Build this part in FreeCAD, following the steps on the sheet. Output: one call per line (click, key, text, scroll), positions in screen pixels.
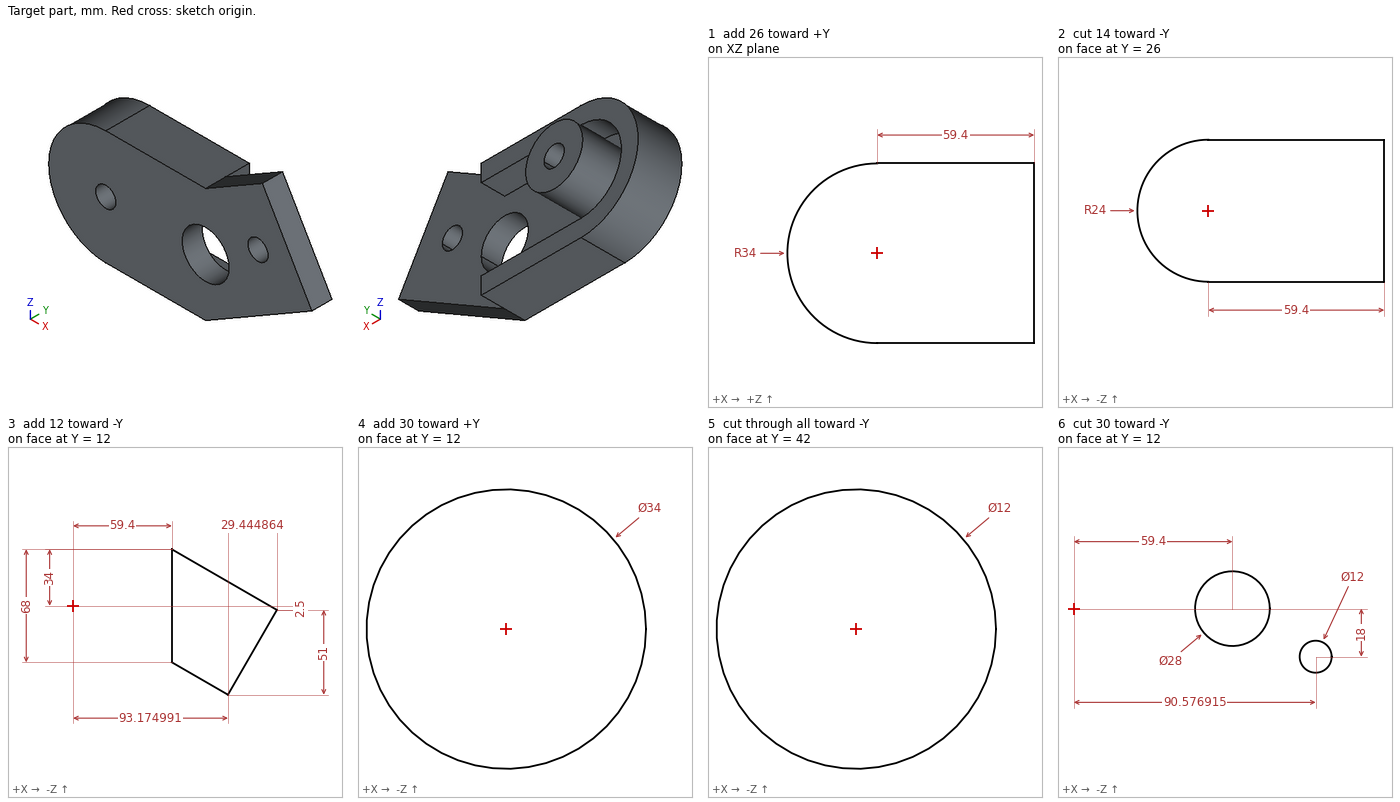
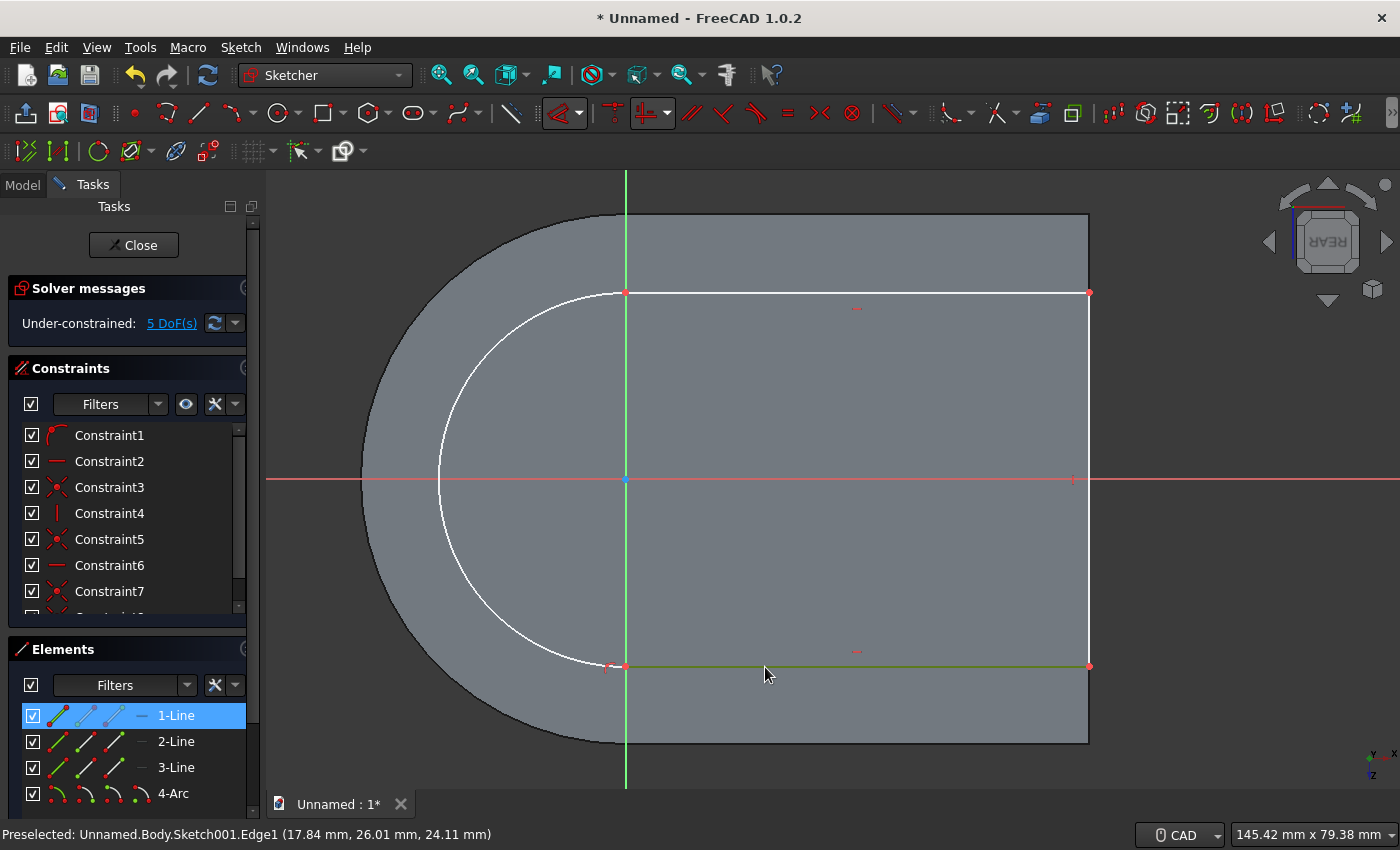
click(475, 370)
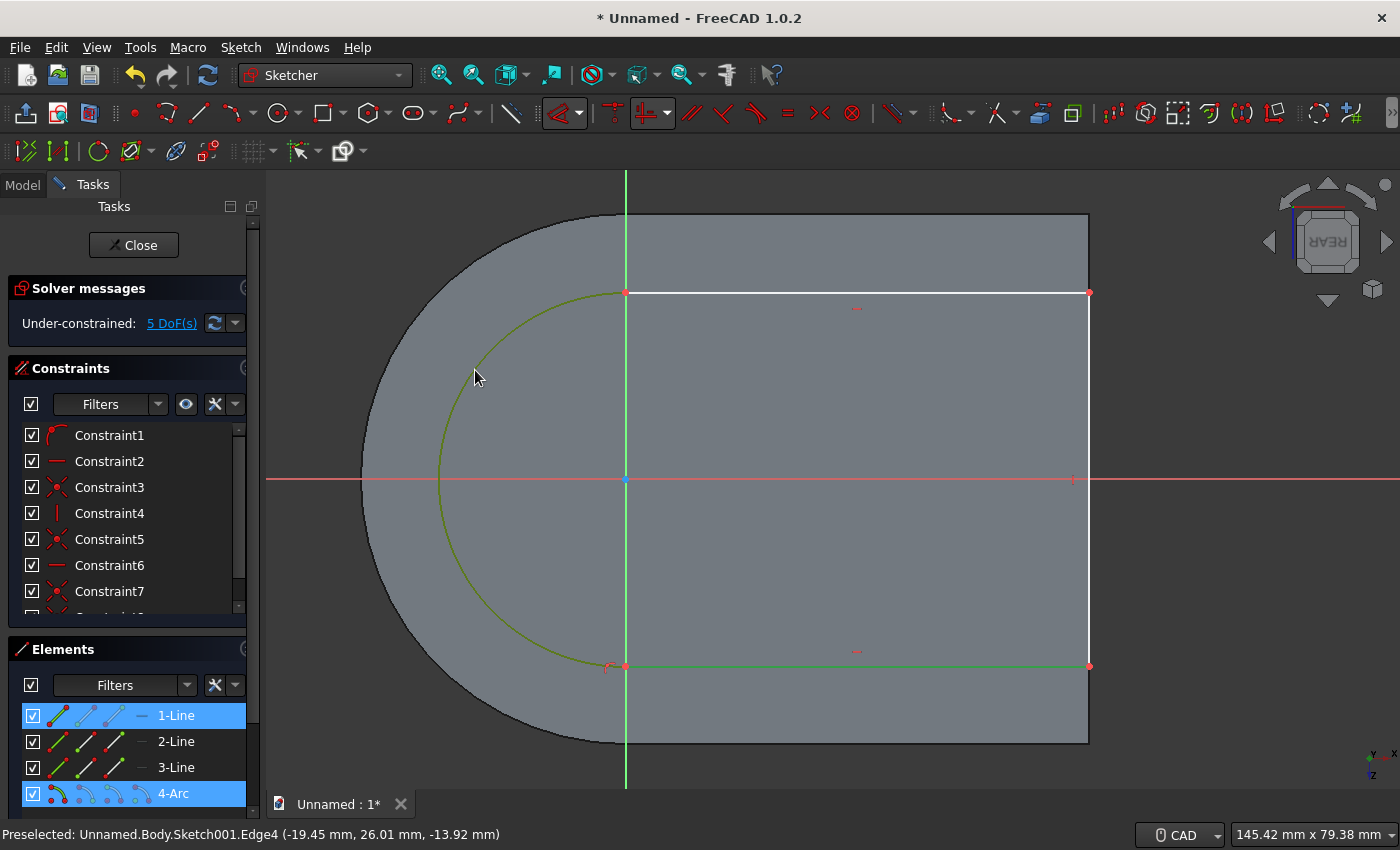
click(756, 114)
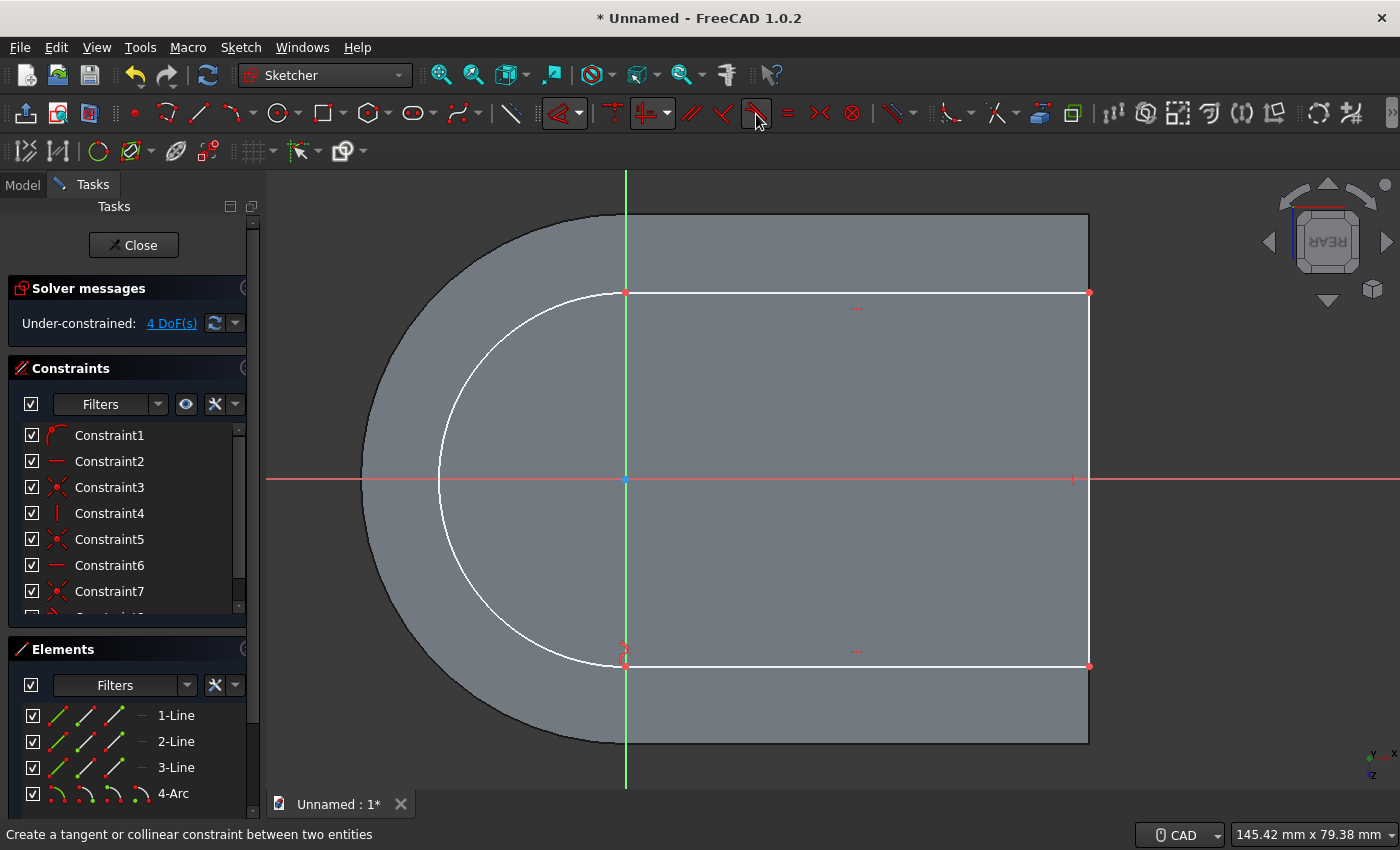
click(950, 293)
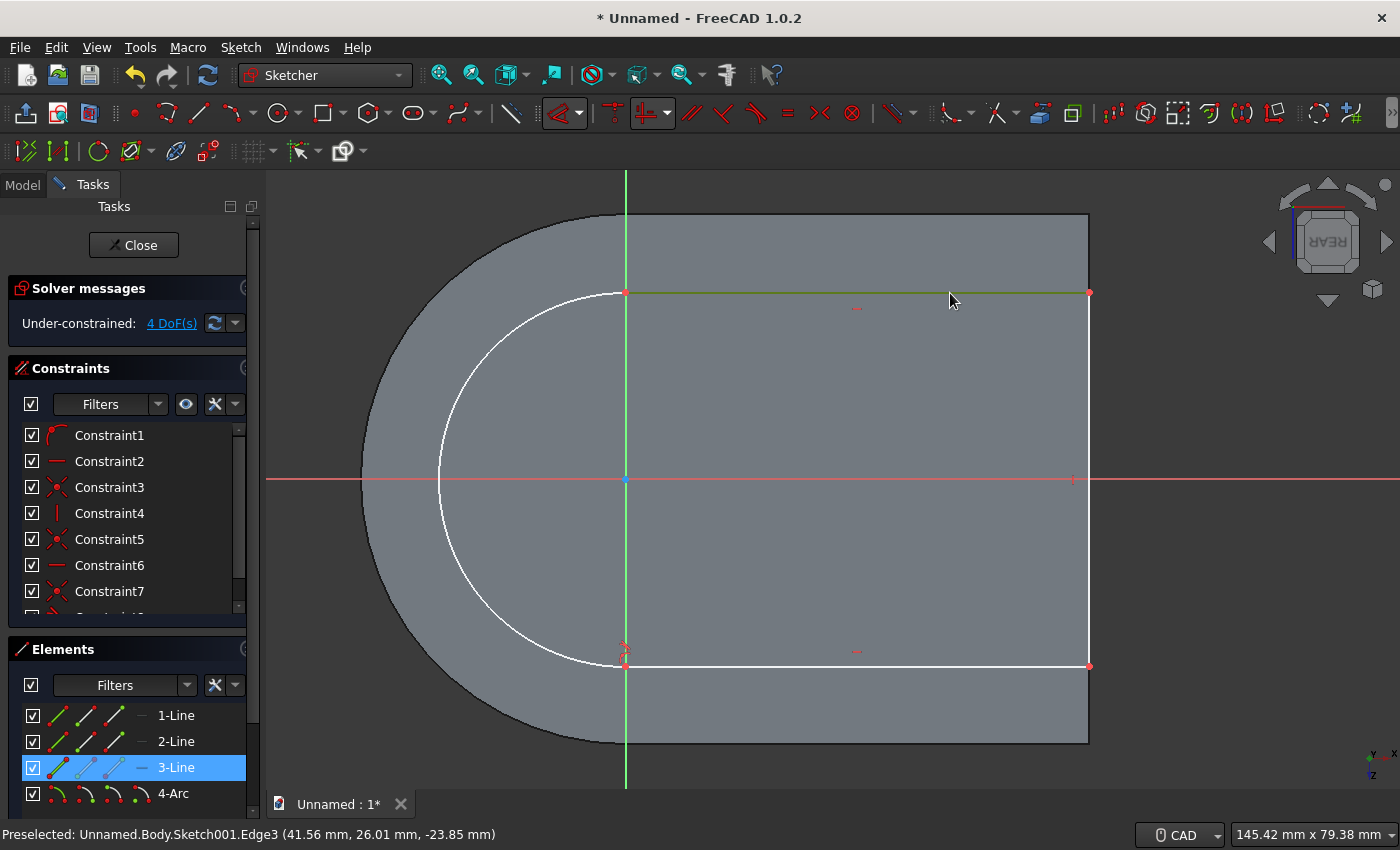
click(475, 370)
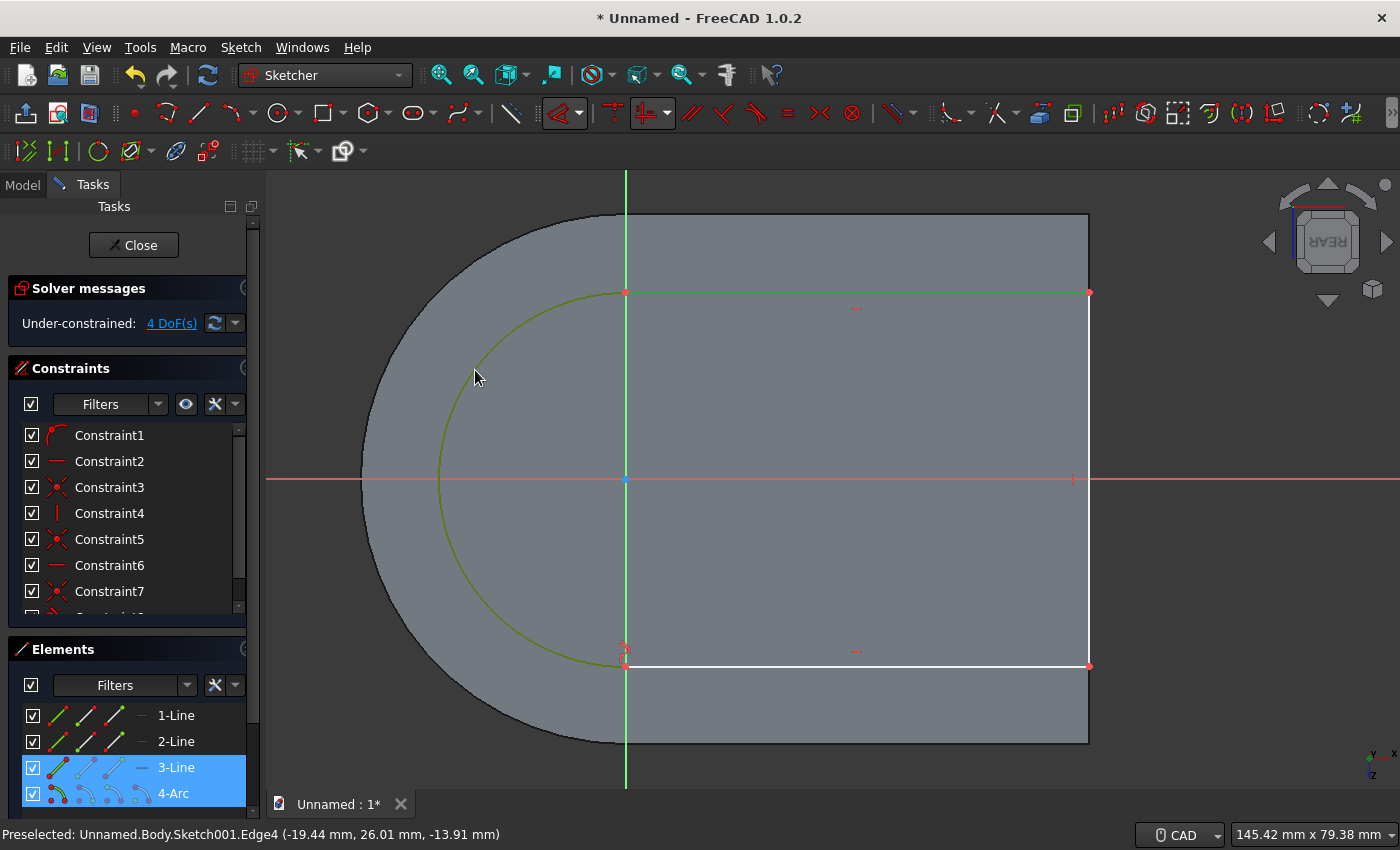
click(756, 114)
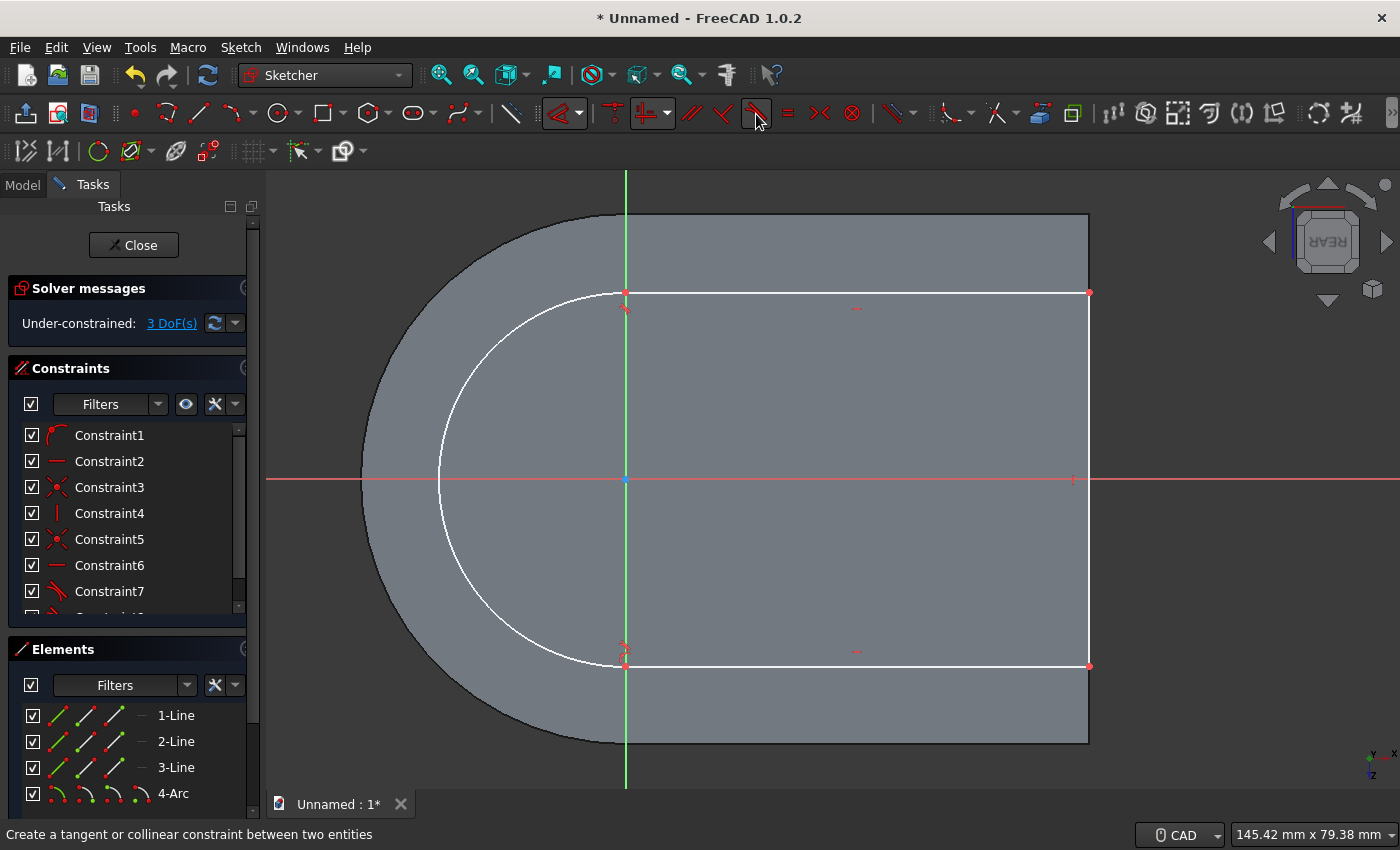
click(626, 480)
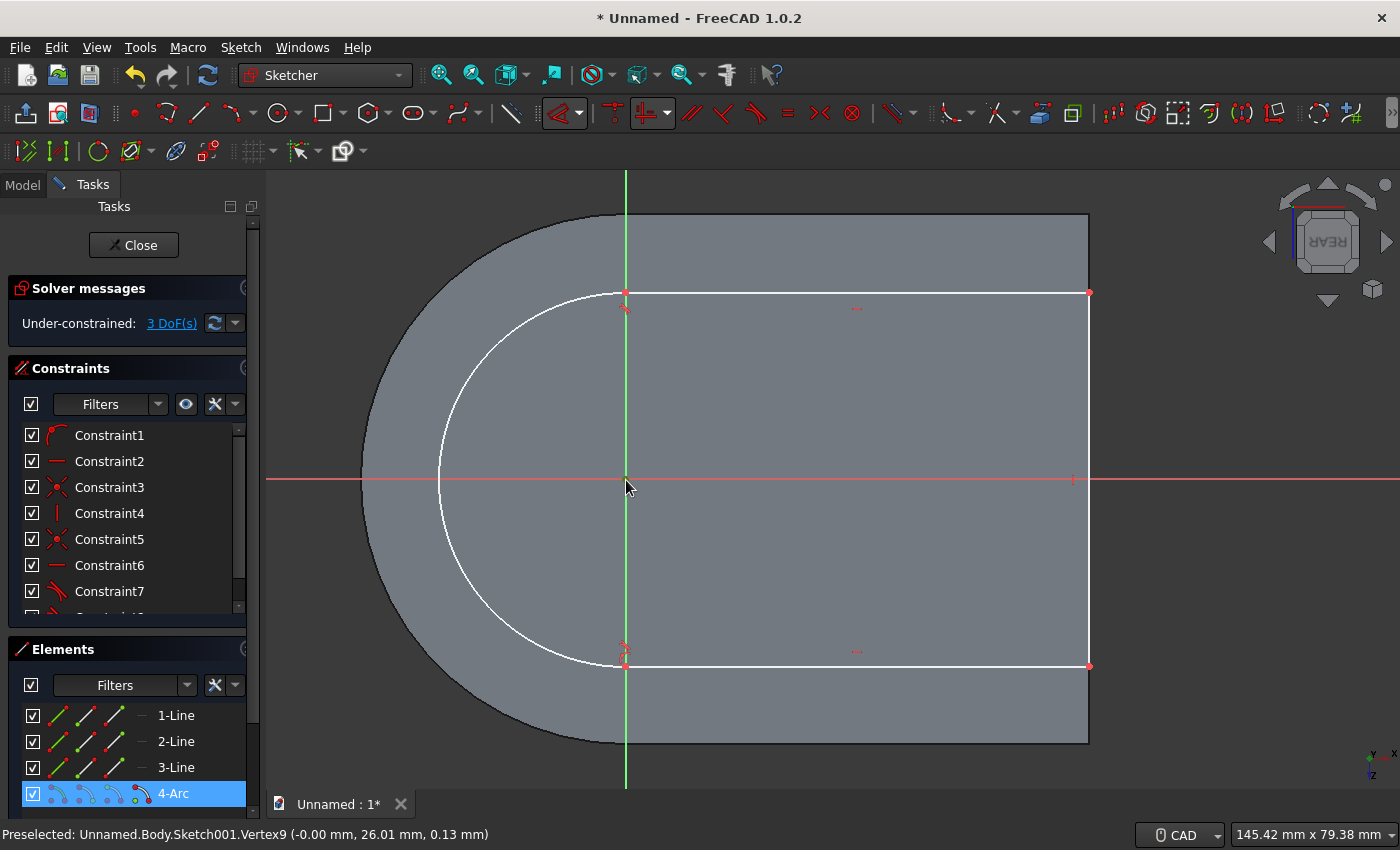
click(361, 479)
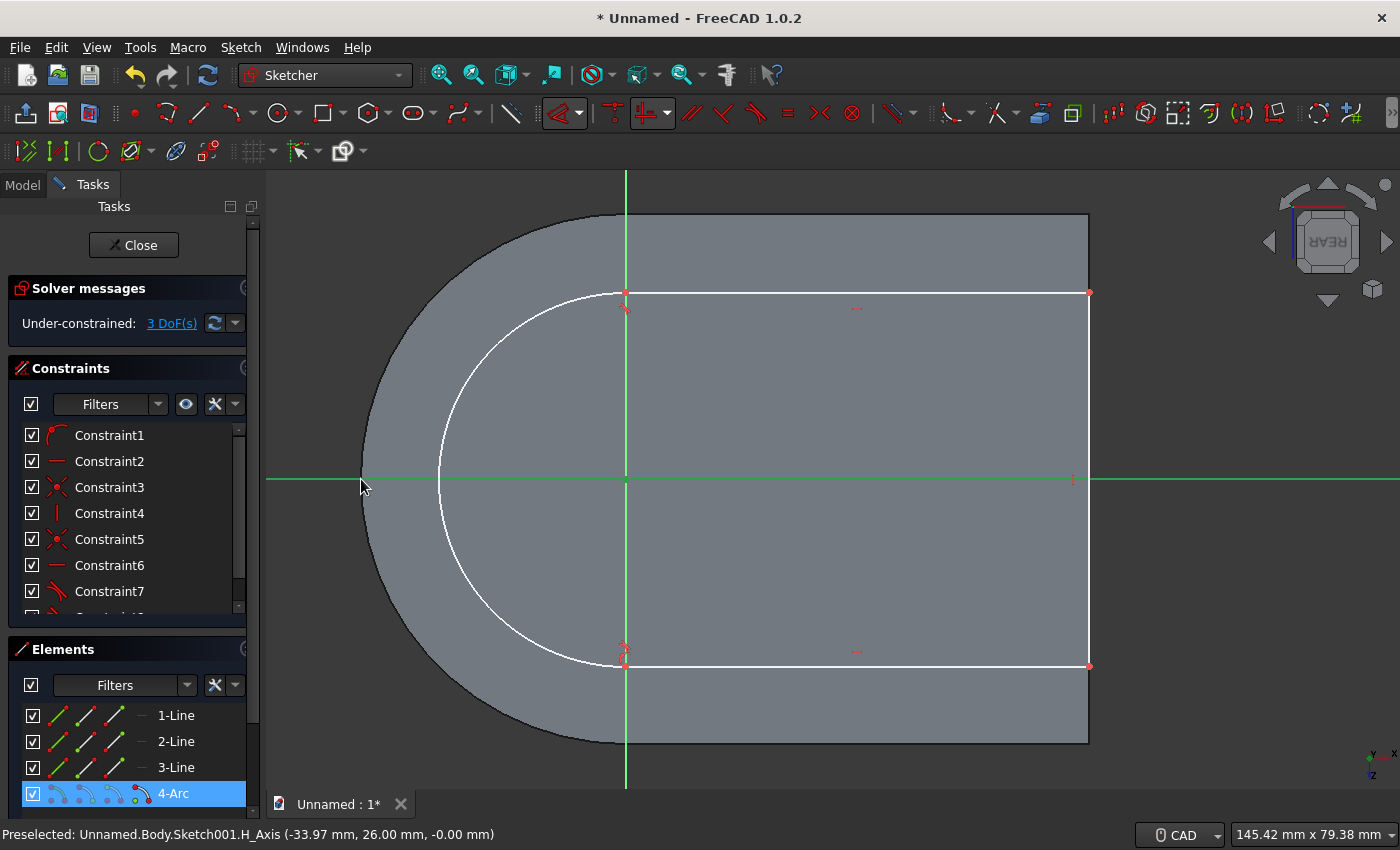
click(614, 114)